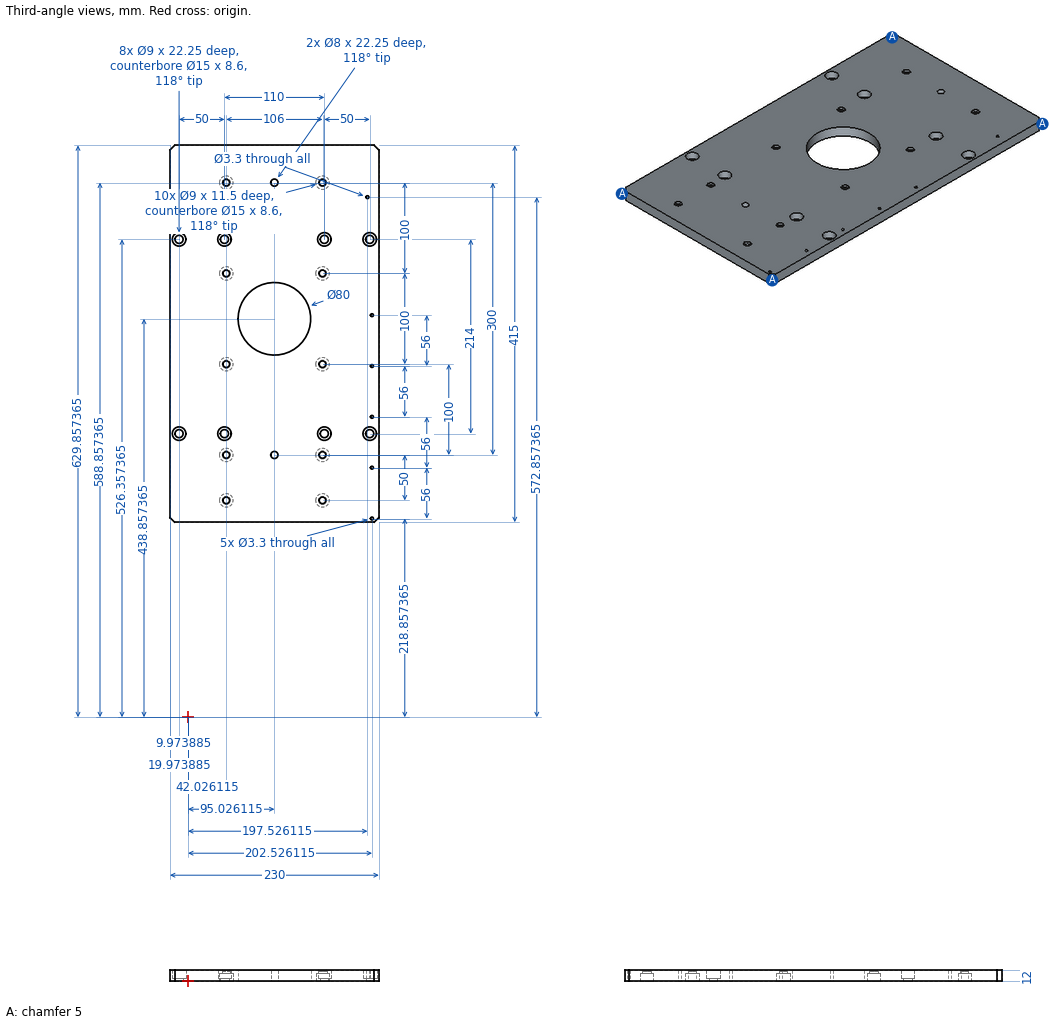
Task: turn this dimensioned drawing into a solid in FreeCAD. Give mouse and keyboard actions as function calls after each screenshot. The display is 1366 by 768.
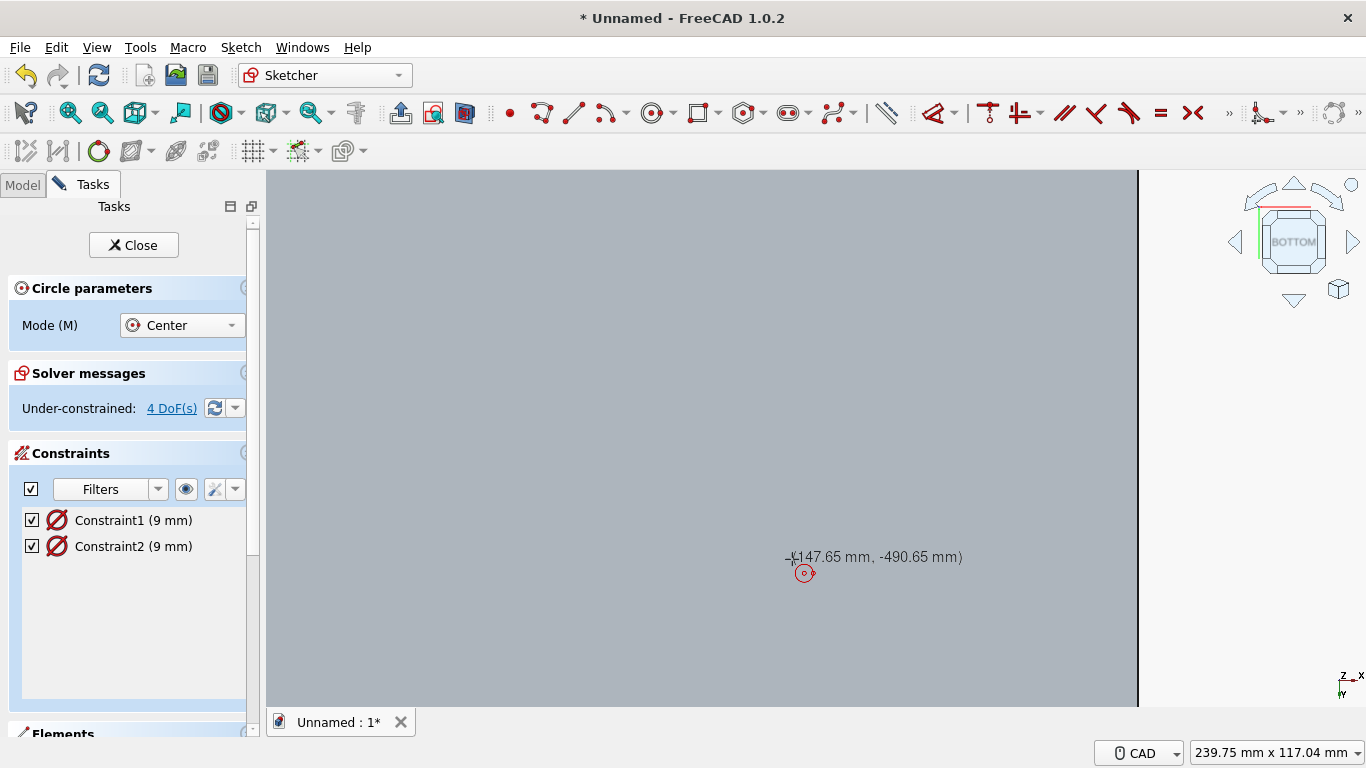
scroll(792, 559, down, 11)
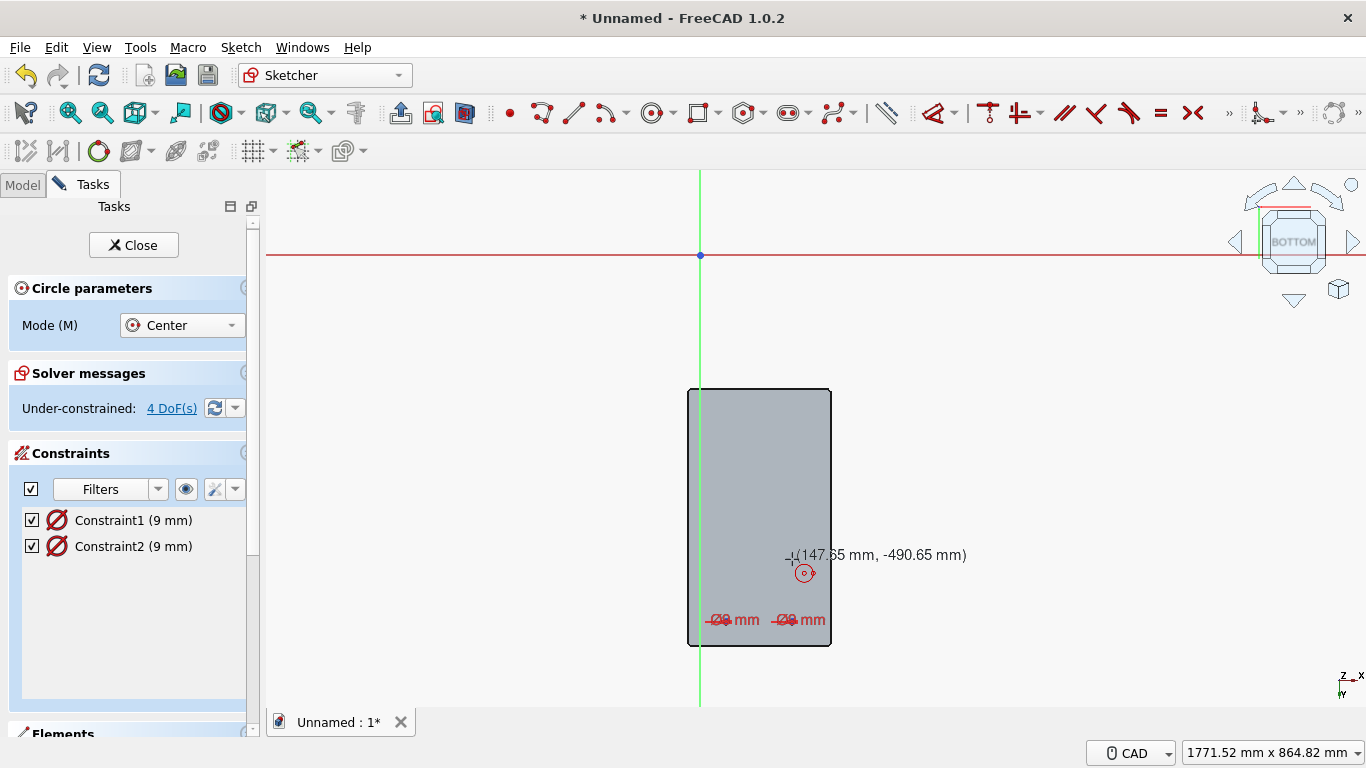
click(792, 559)
move(794, 557)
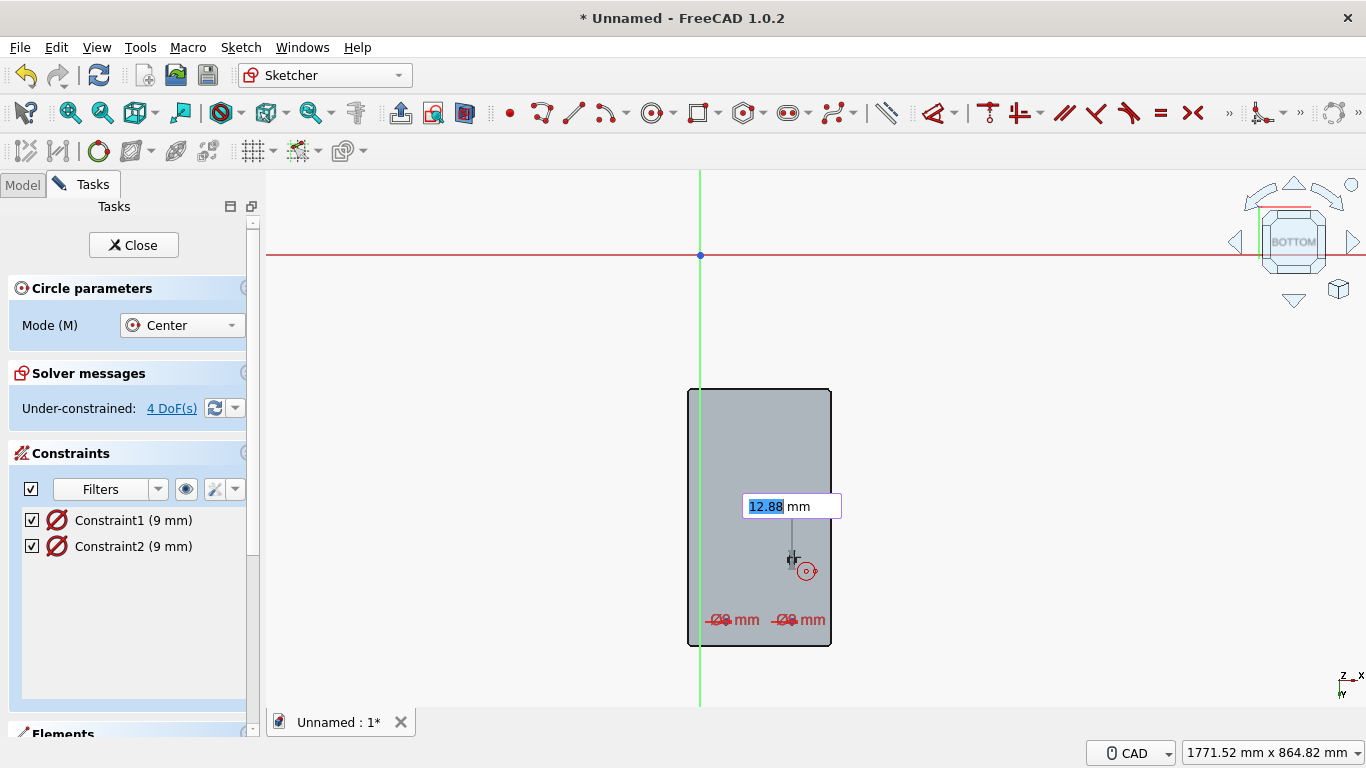
text(9)
key(Return)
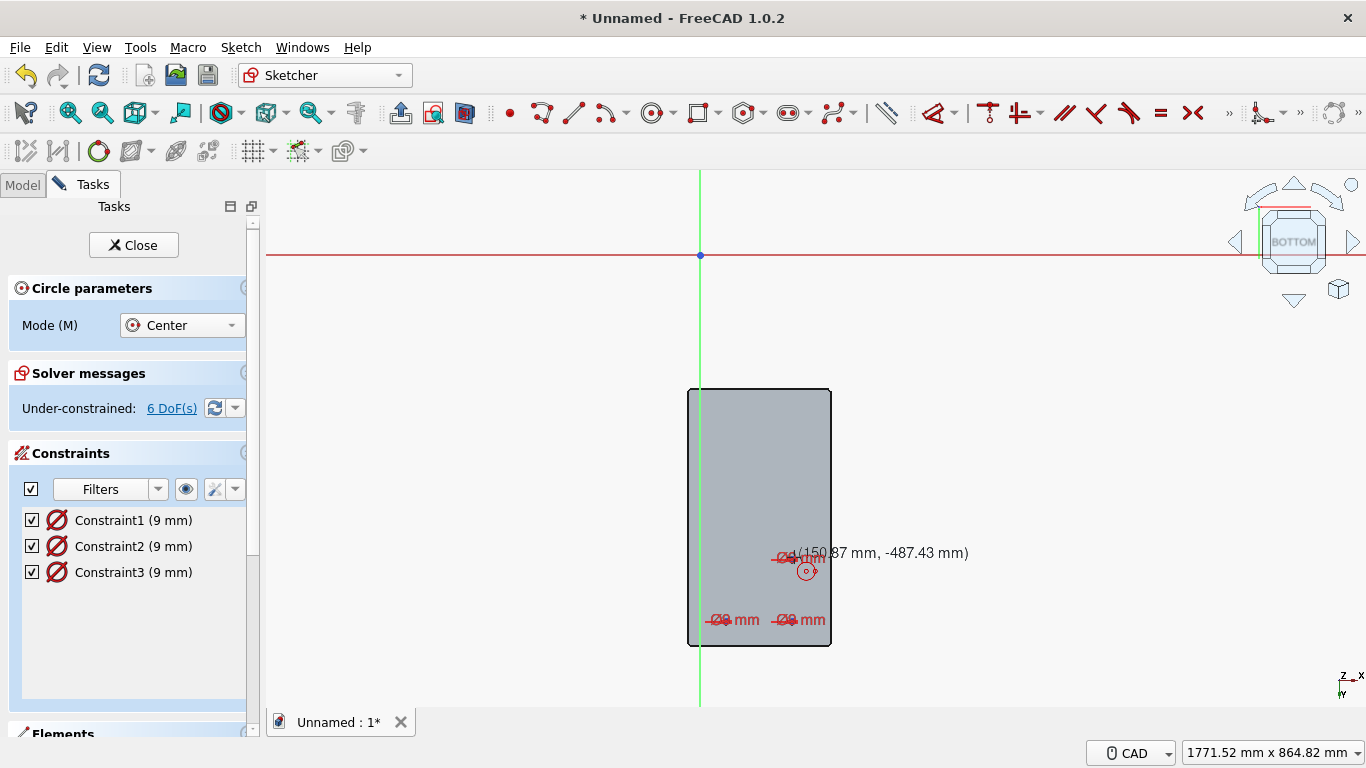
scroll(726, 559, up, 11)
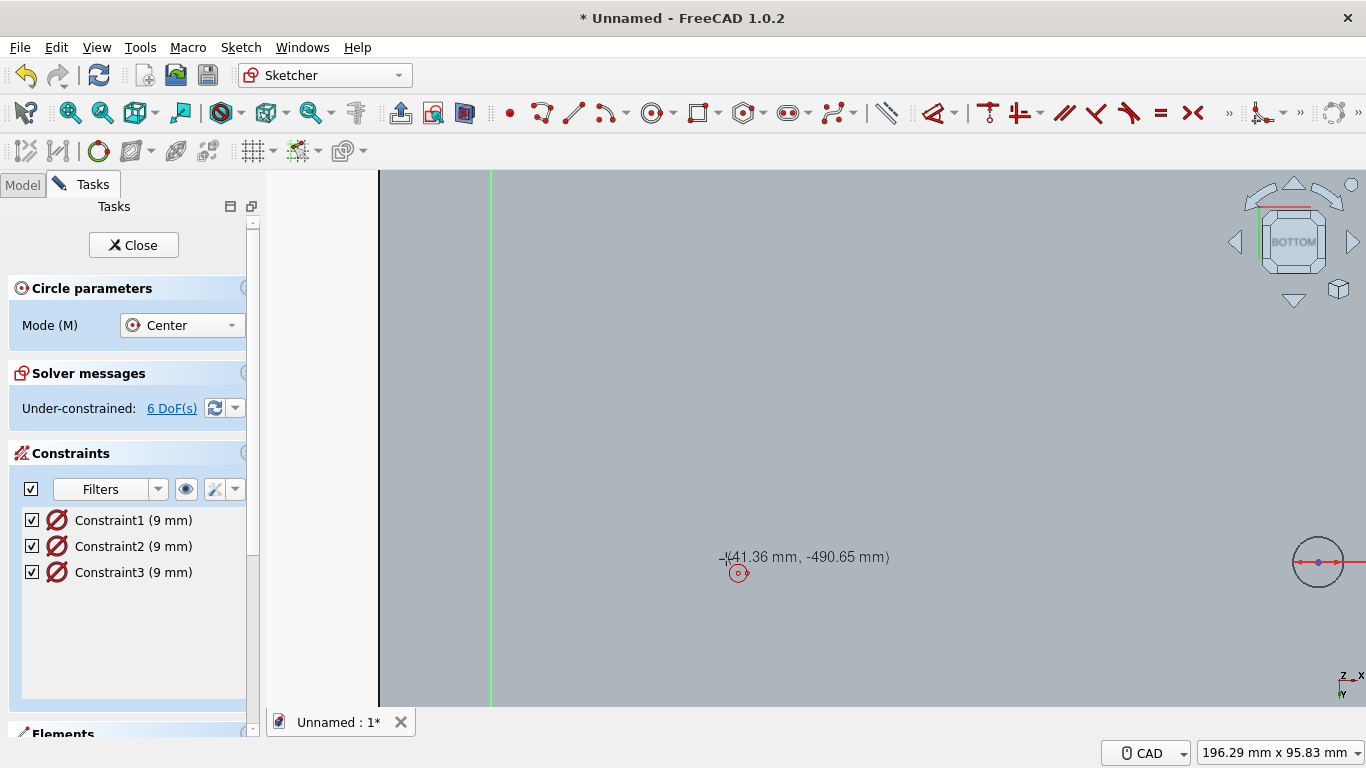
scroll(726, 559, down, 11)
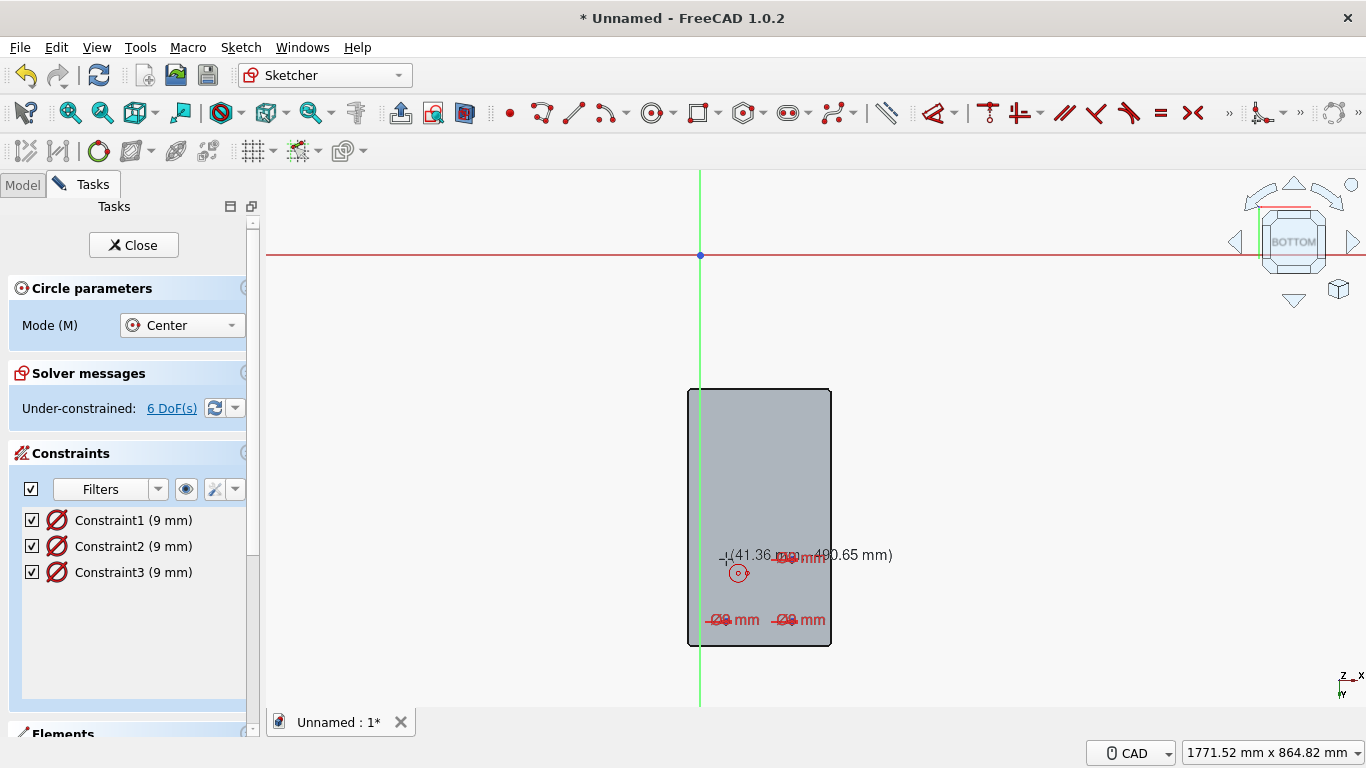
click(726, 559)
move(728, 557)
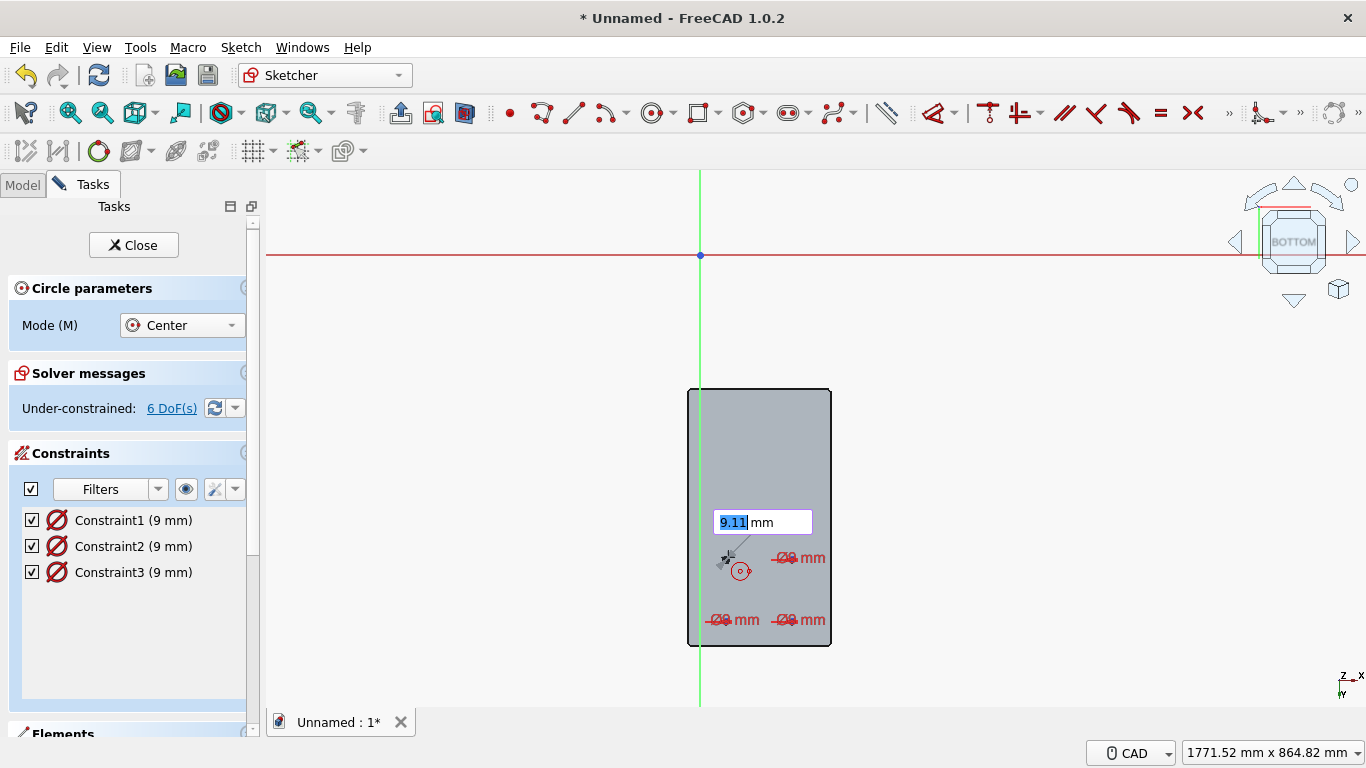
text(9)
key(Return)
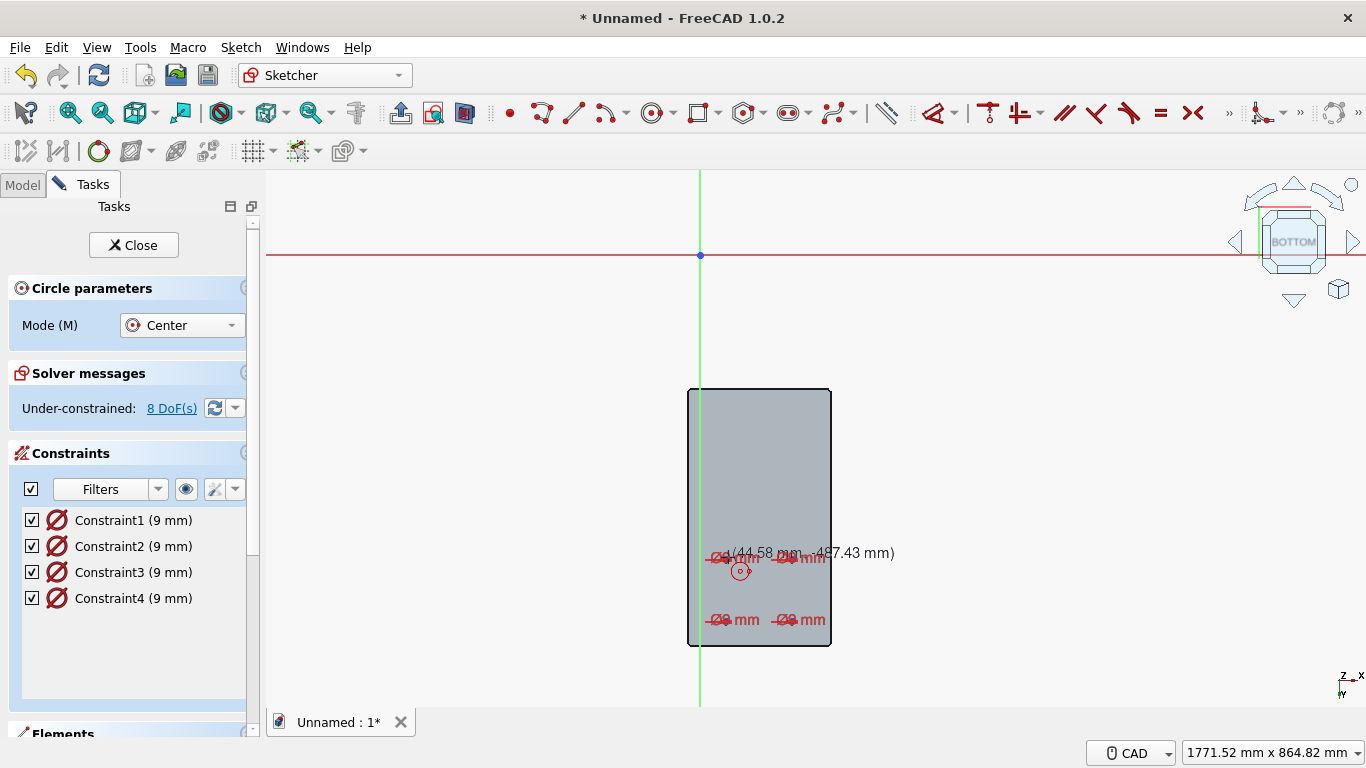
scroll(792, 497, up, 11)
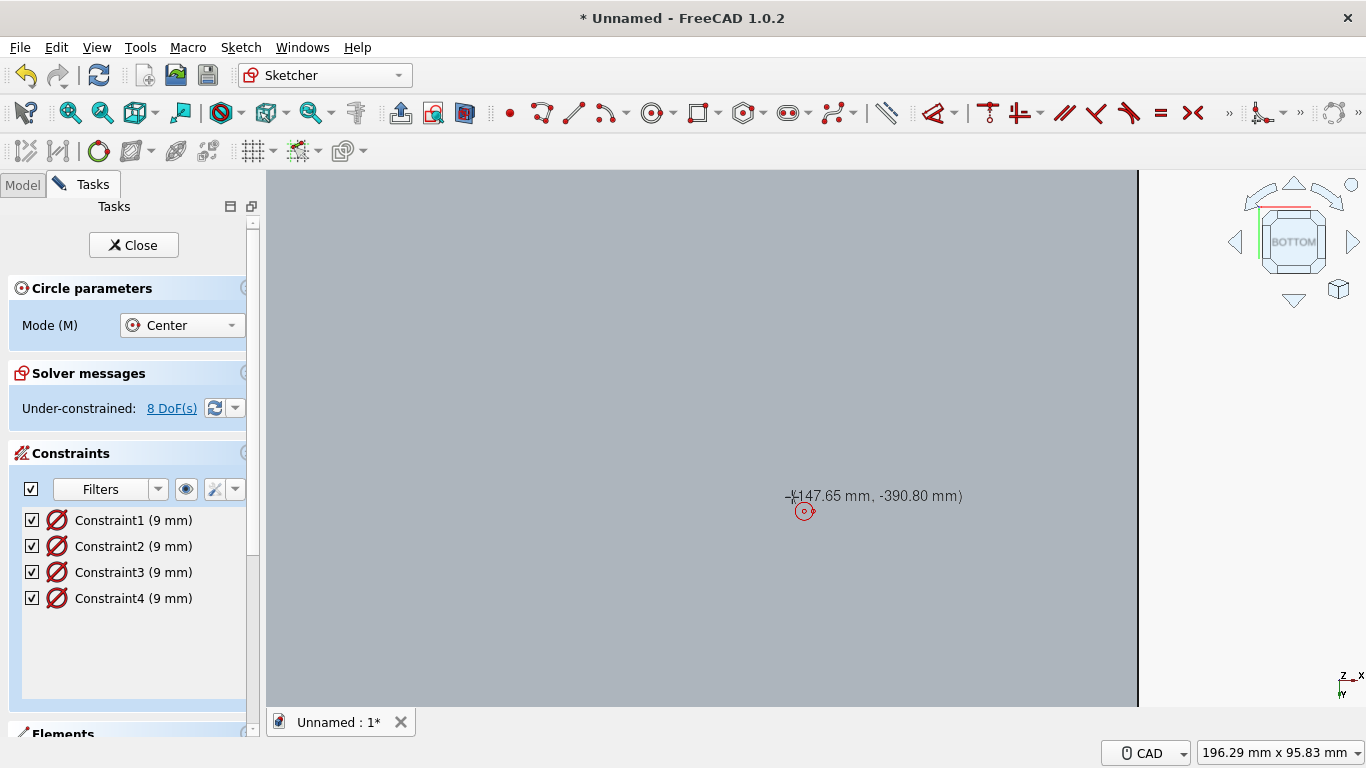
scroll(792, 496, down, 11)